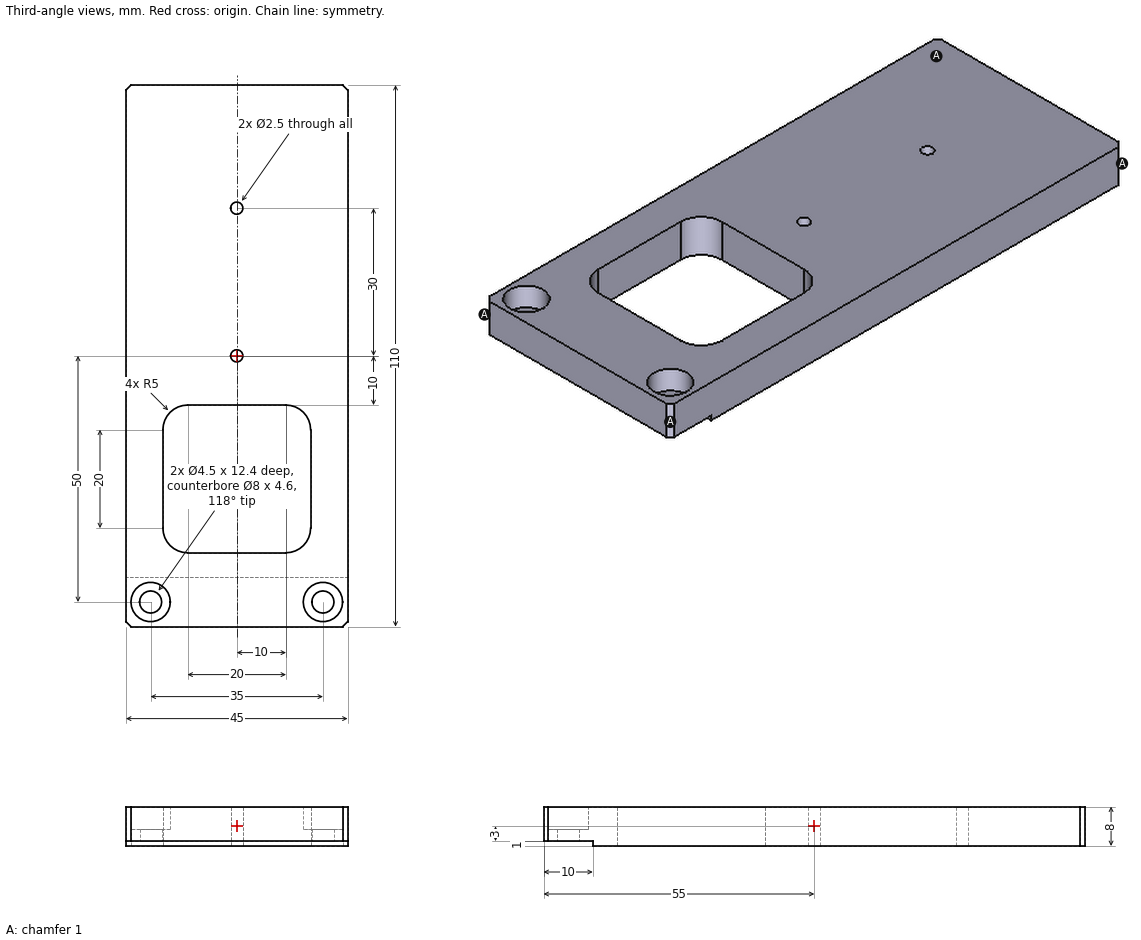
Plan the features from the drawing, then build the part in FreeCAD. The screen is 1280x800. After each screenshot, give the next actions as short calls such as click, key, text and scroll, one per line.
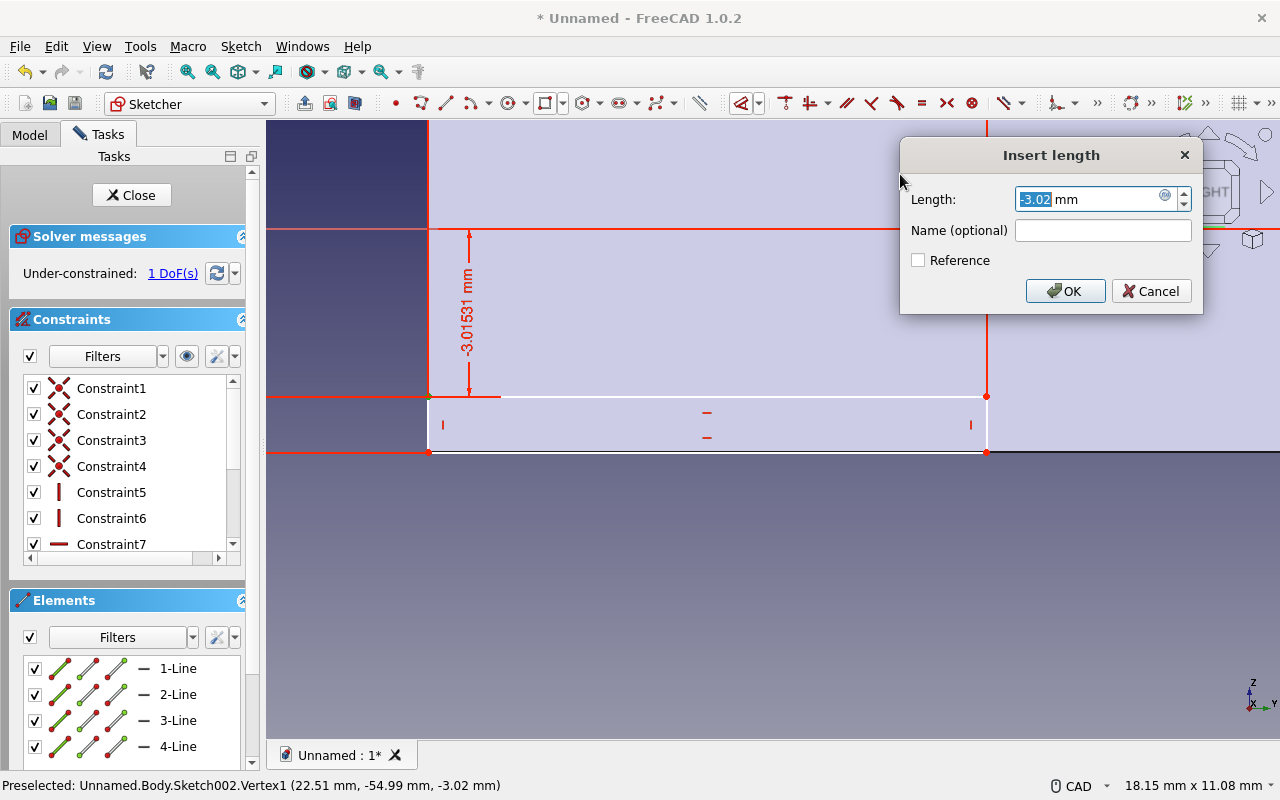
text(-3)
key(Return)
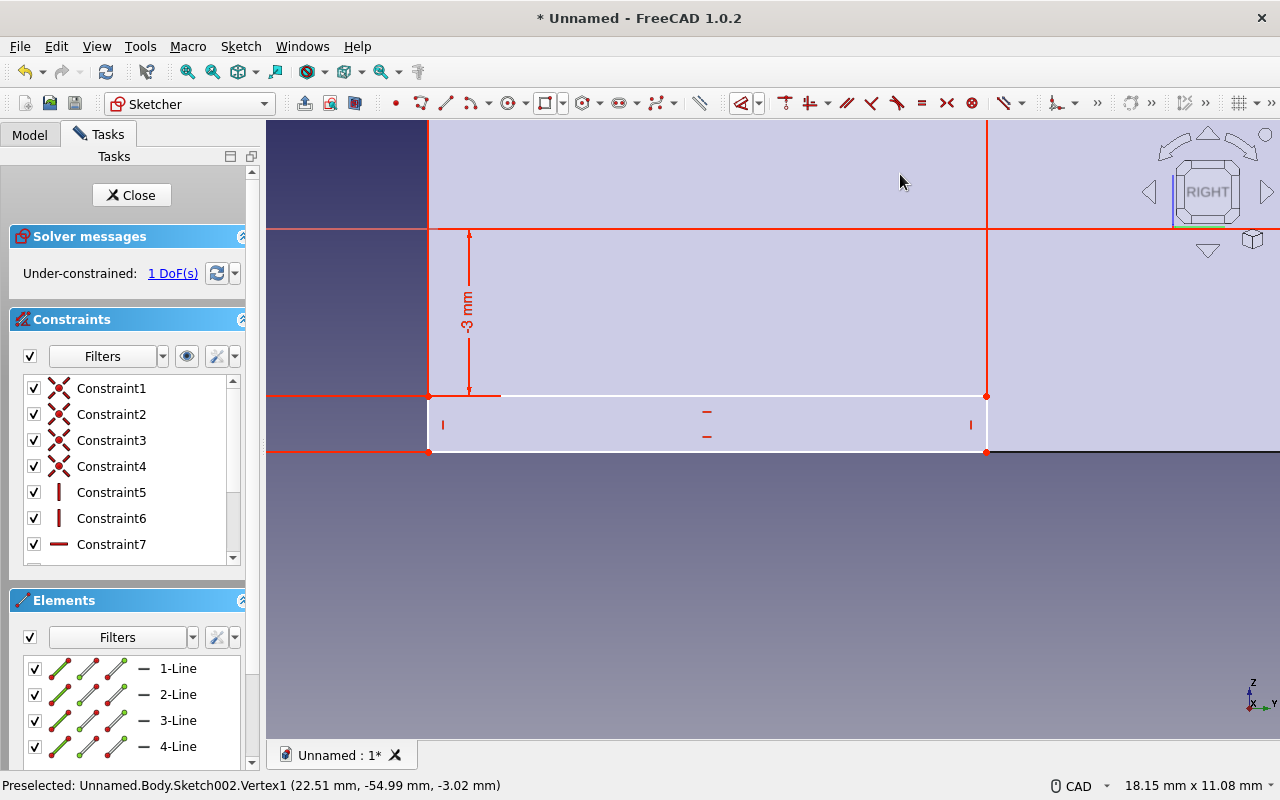
click(428, 396)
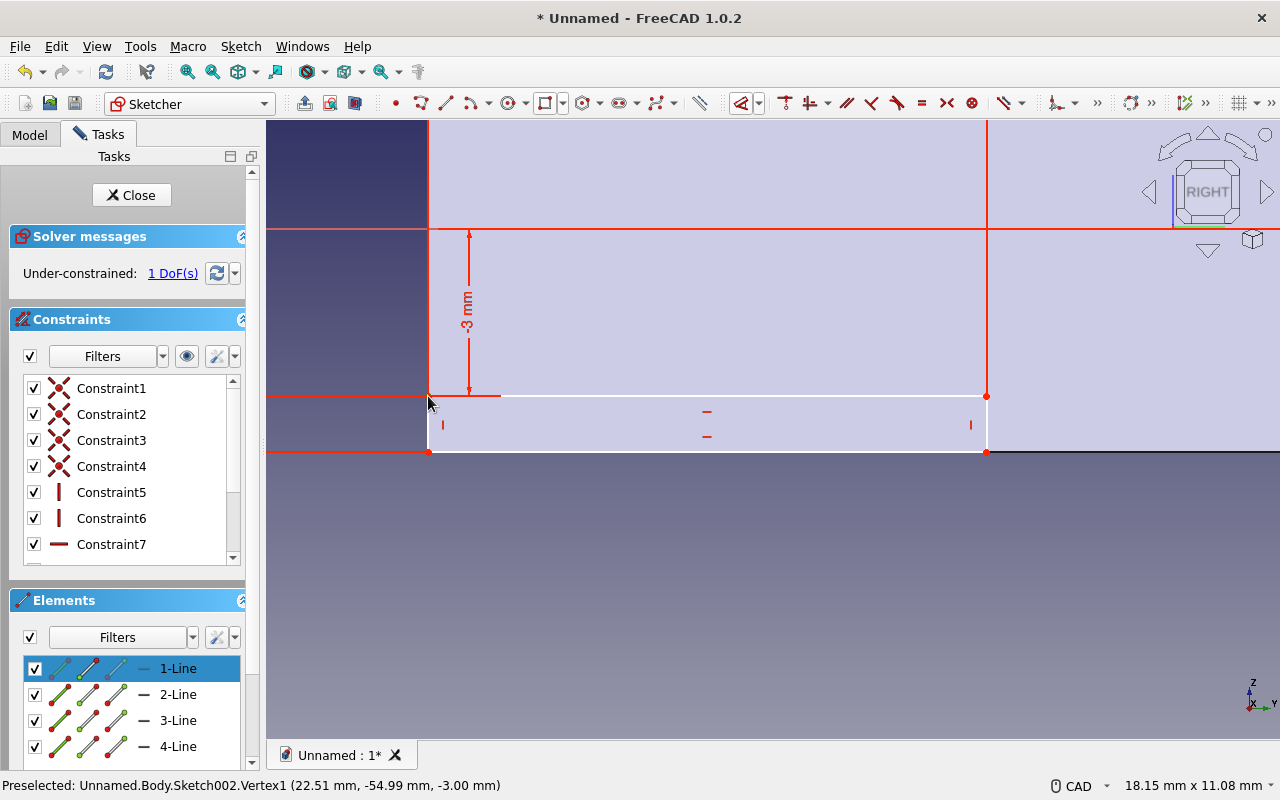
click(758, 104)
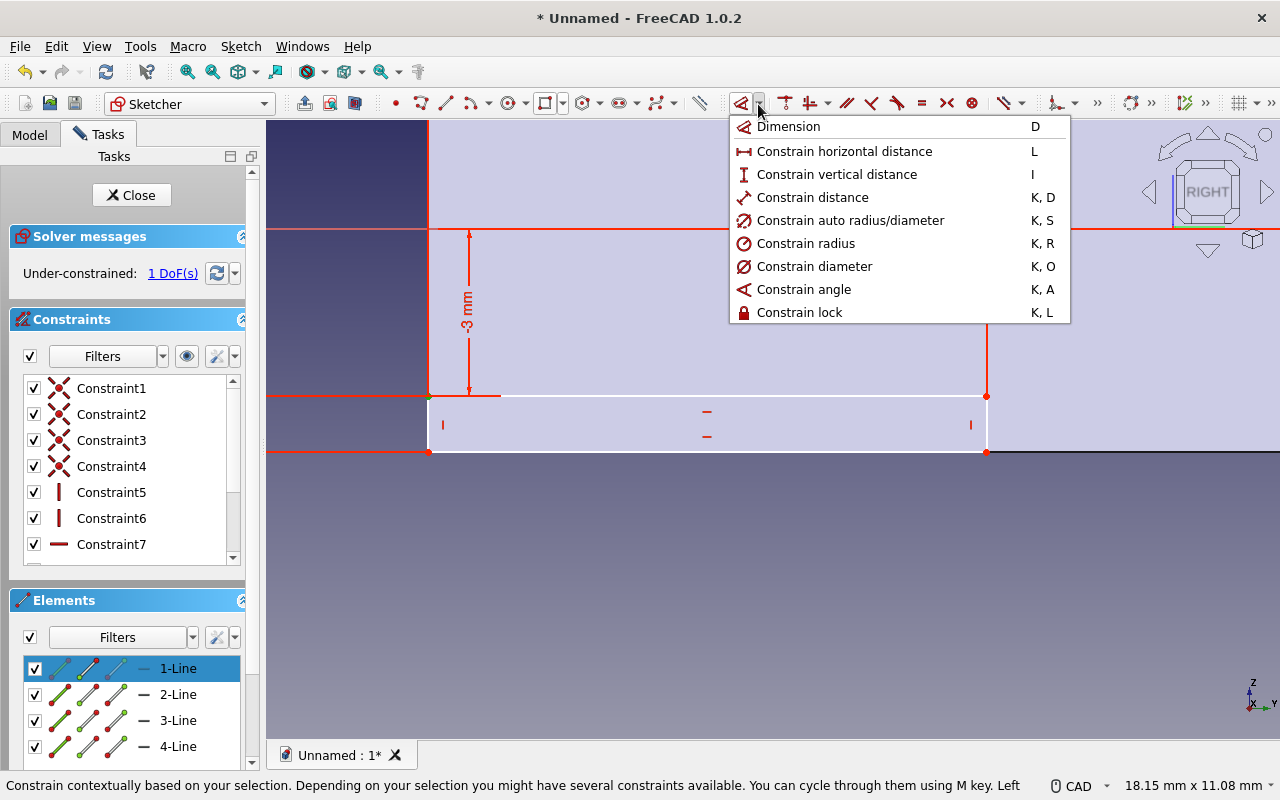
click(900, 152)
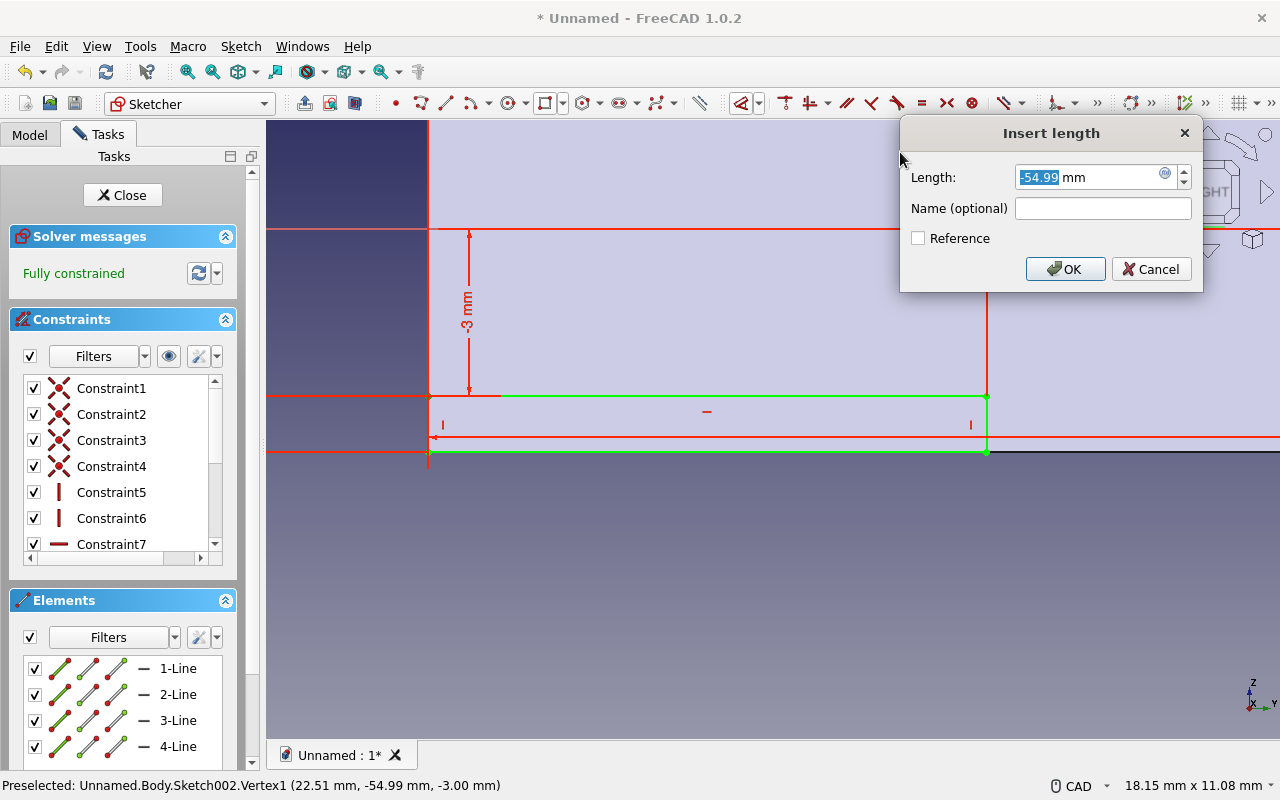
text(-55)
key(Return)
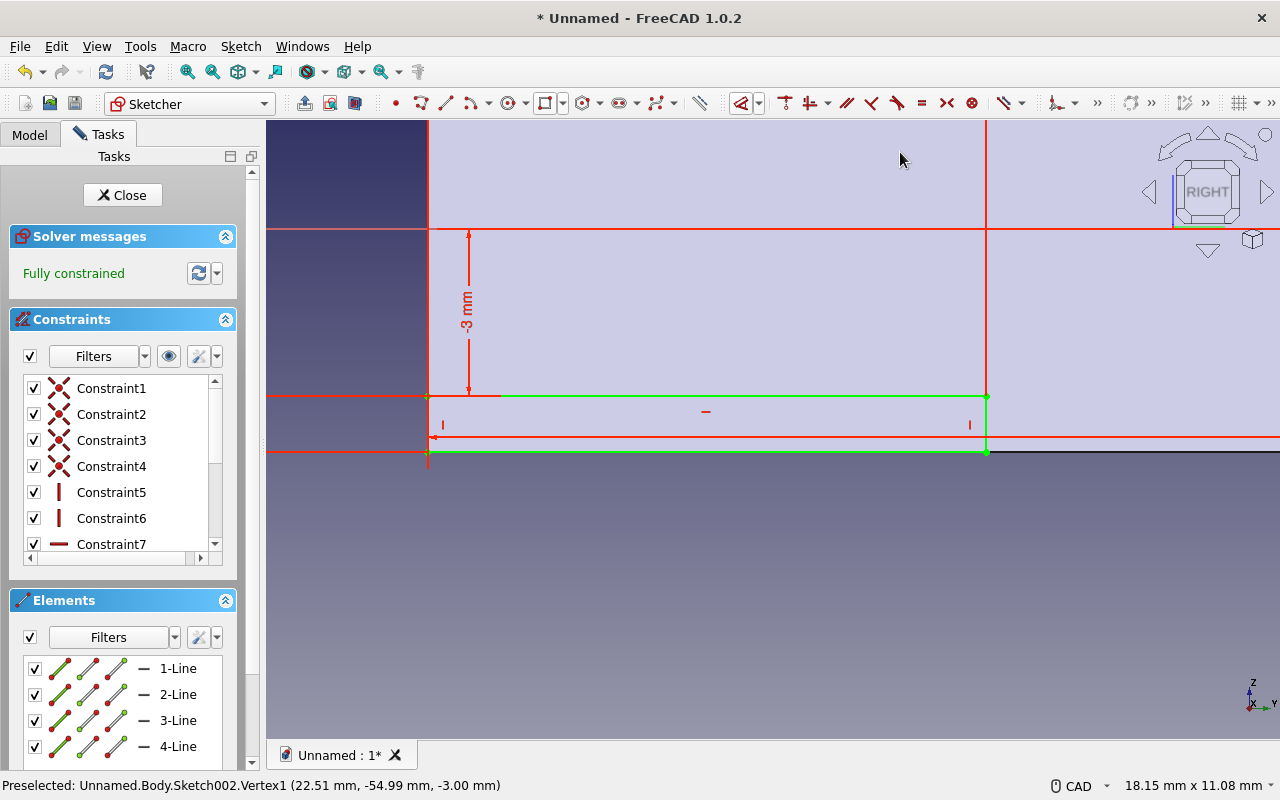
click(123, 195)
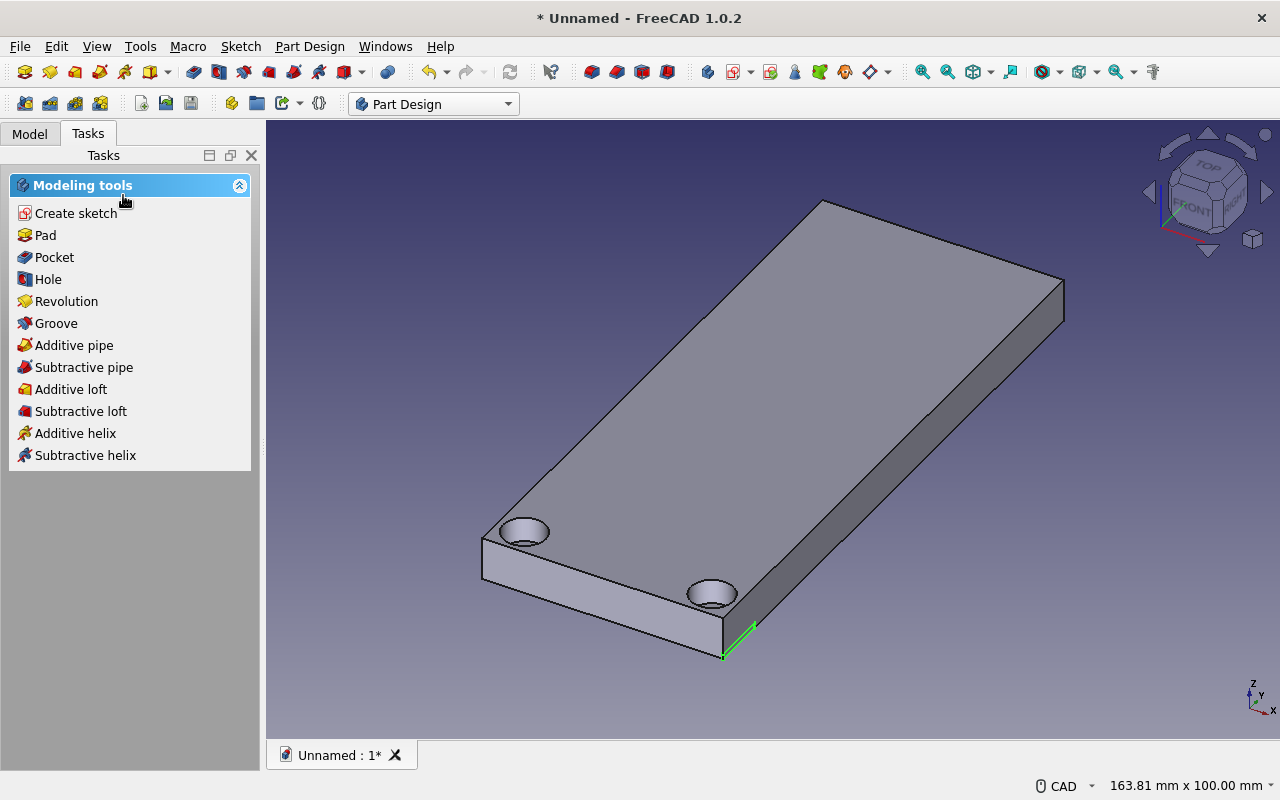
click(194, 72)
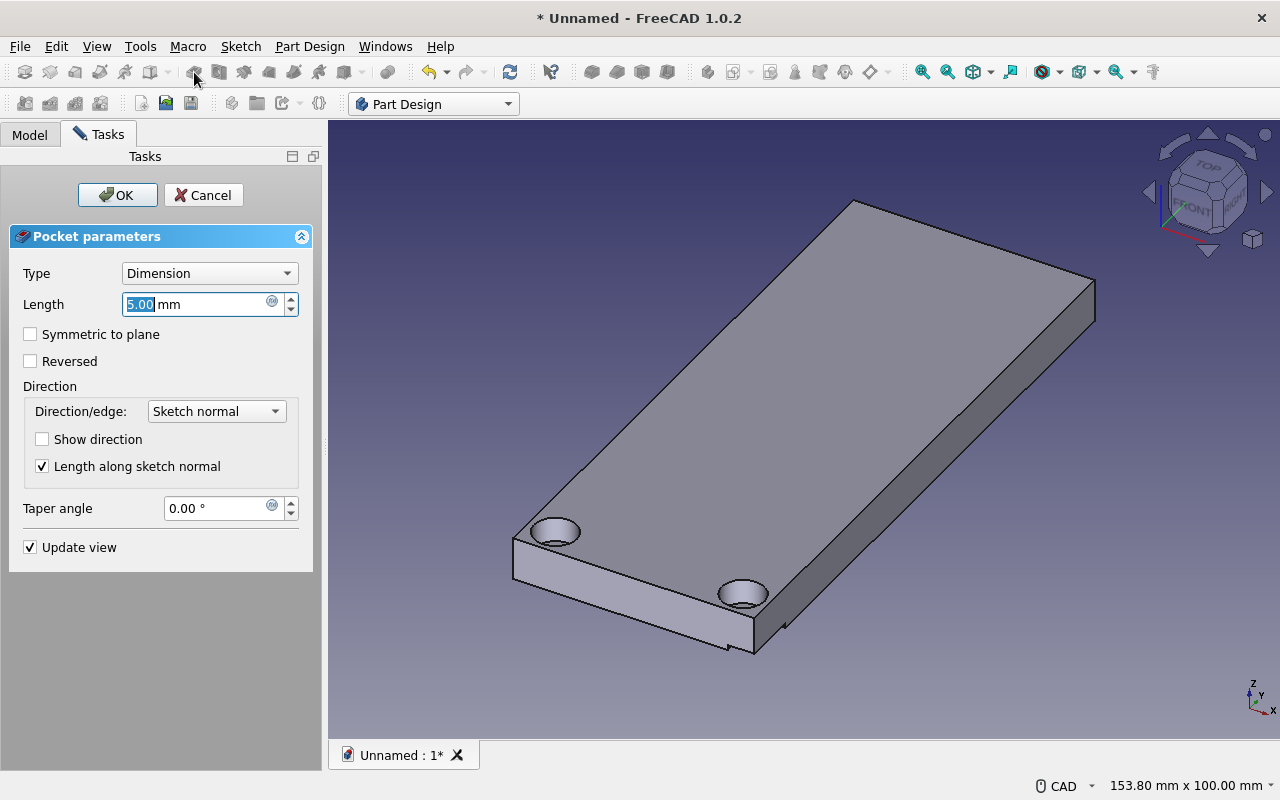
click(210, 274)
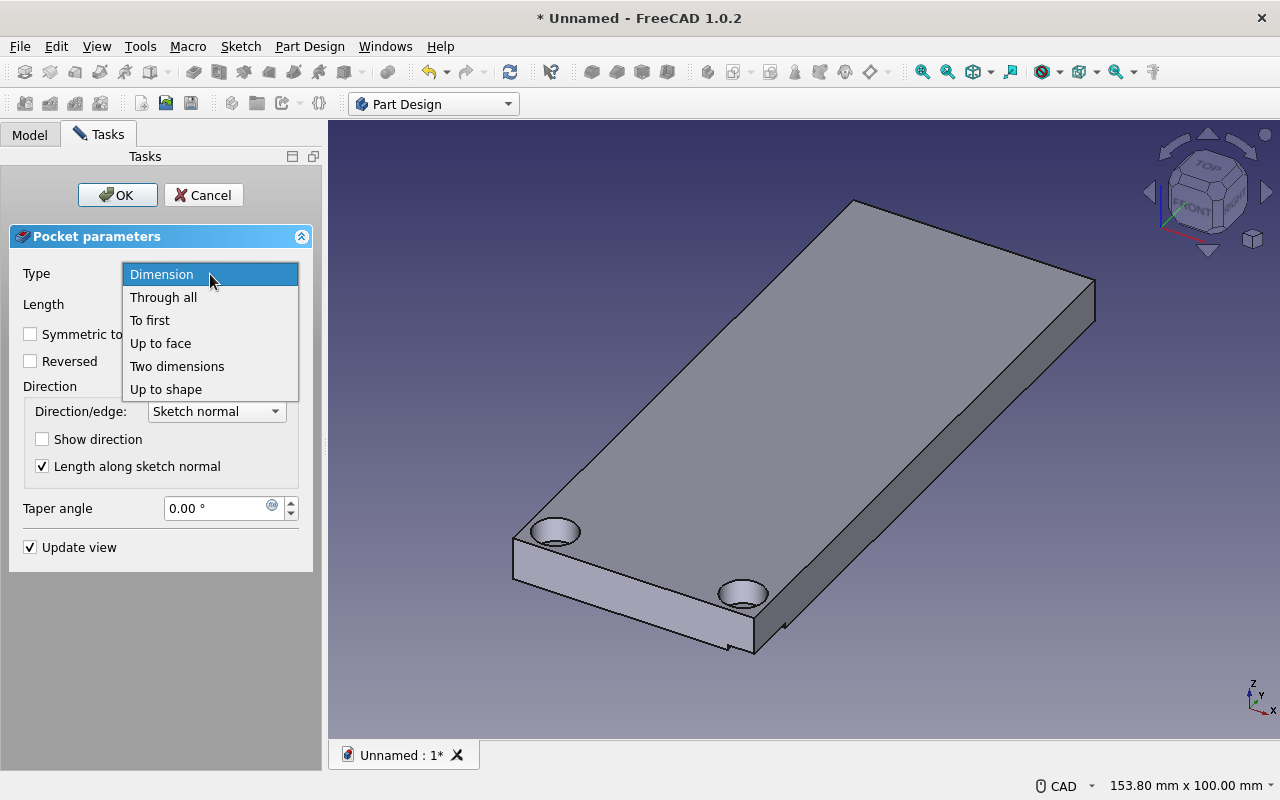
click(208, 298)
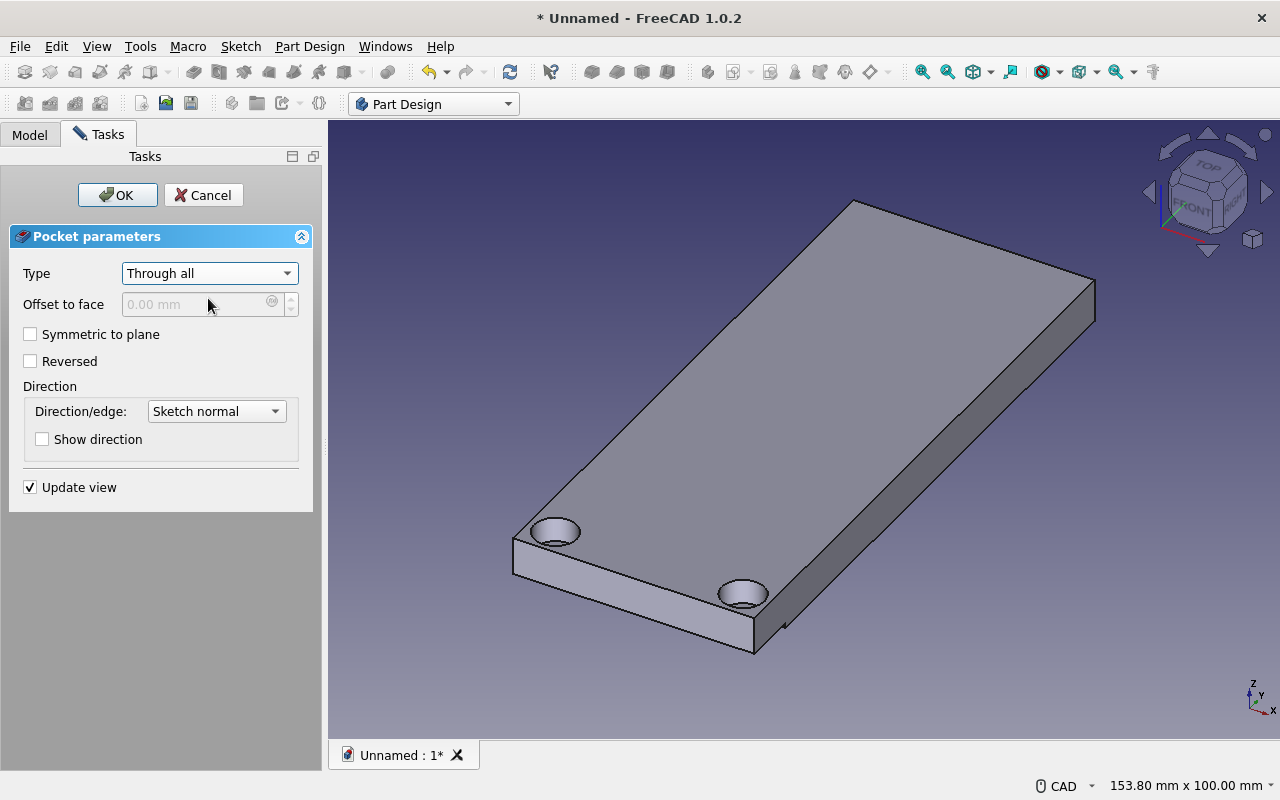
click(118, 195)